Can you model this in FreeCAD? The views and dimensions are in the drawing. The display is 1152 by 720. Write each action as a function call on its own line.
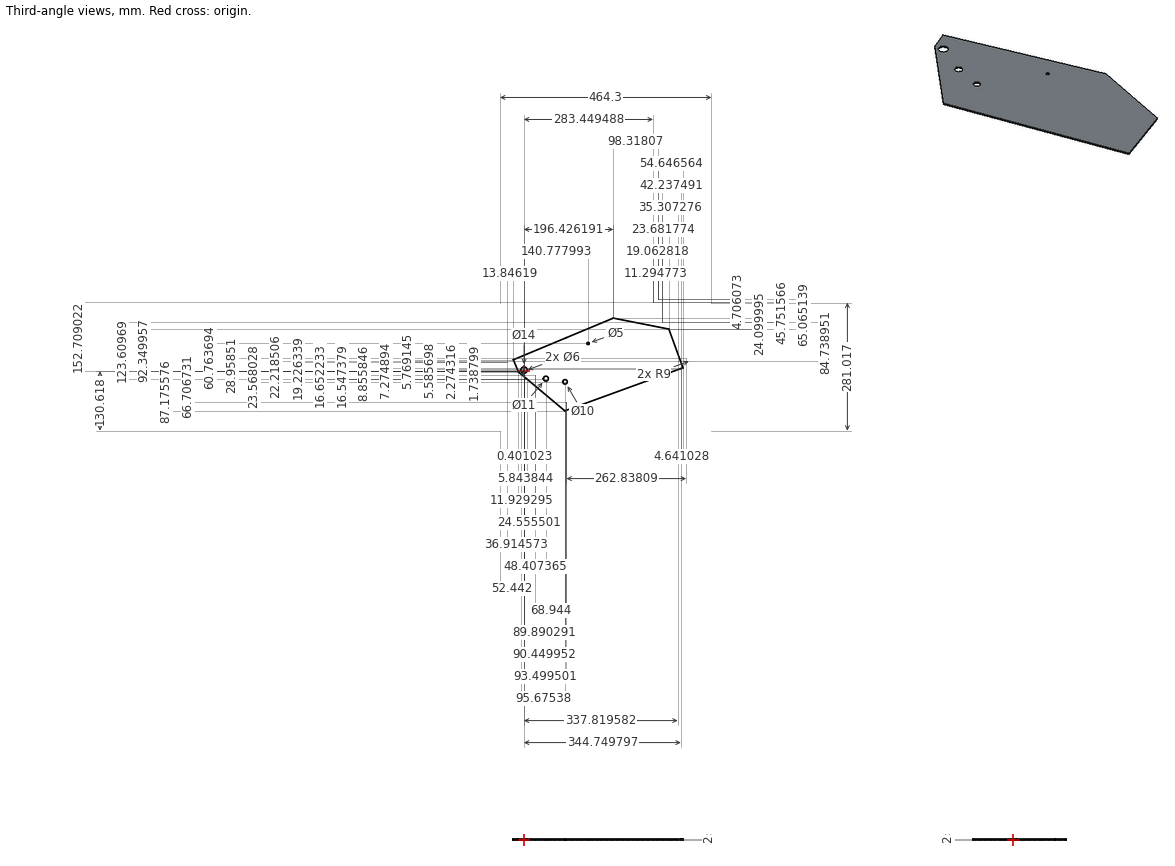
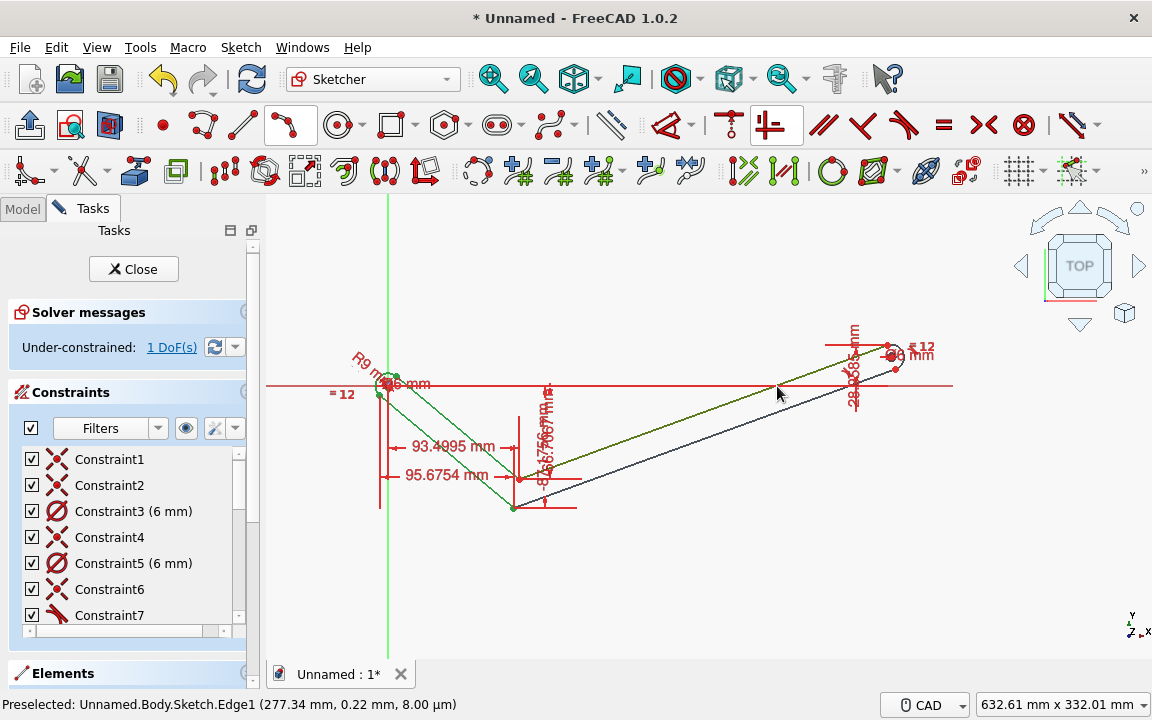
key(l)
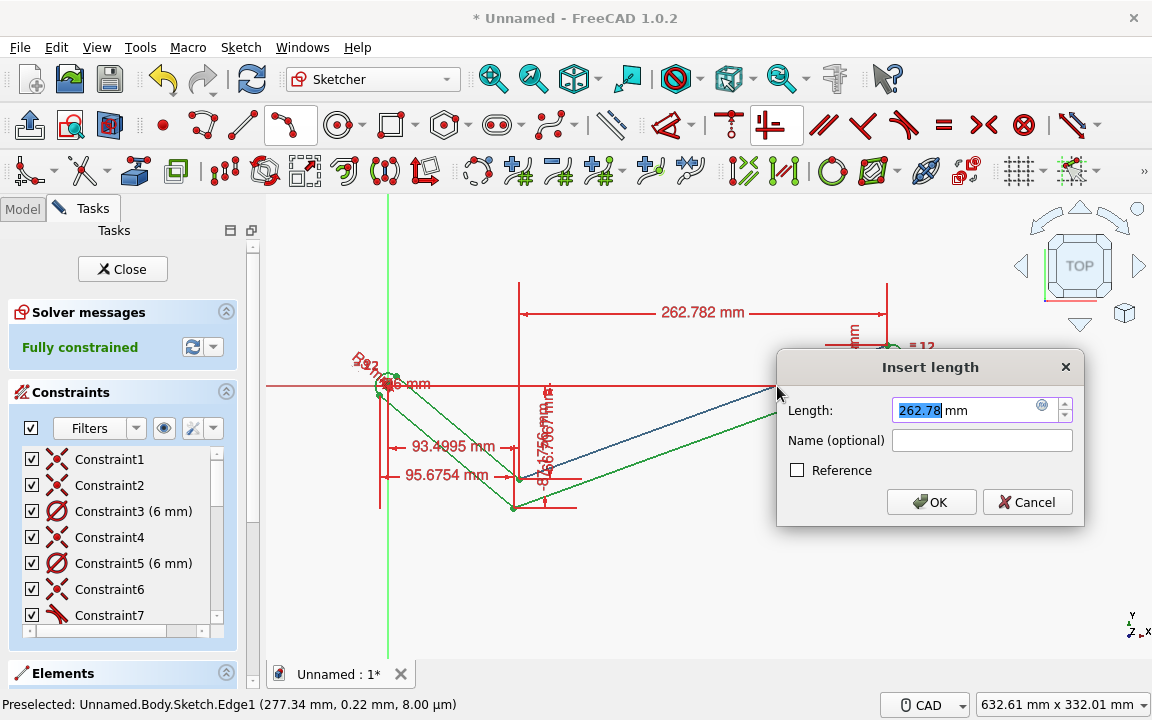
text(262.83809)
key(Return)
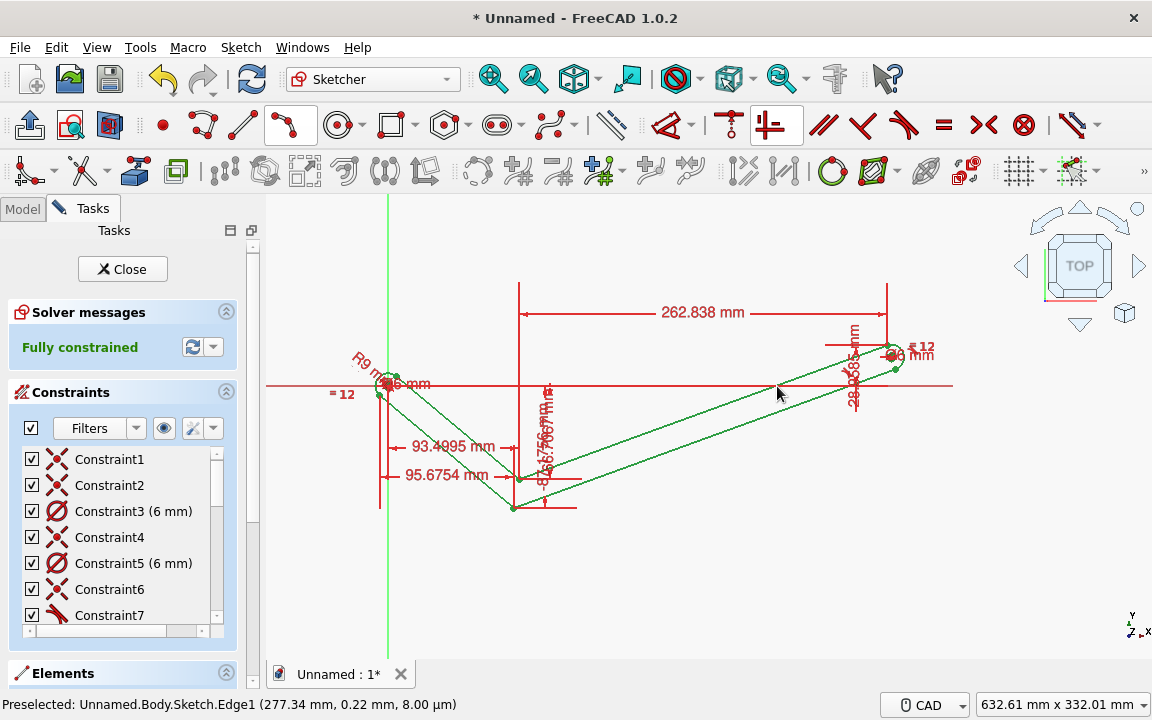
click(123, 269)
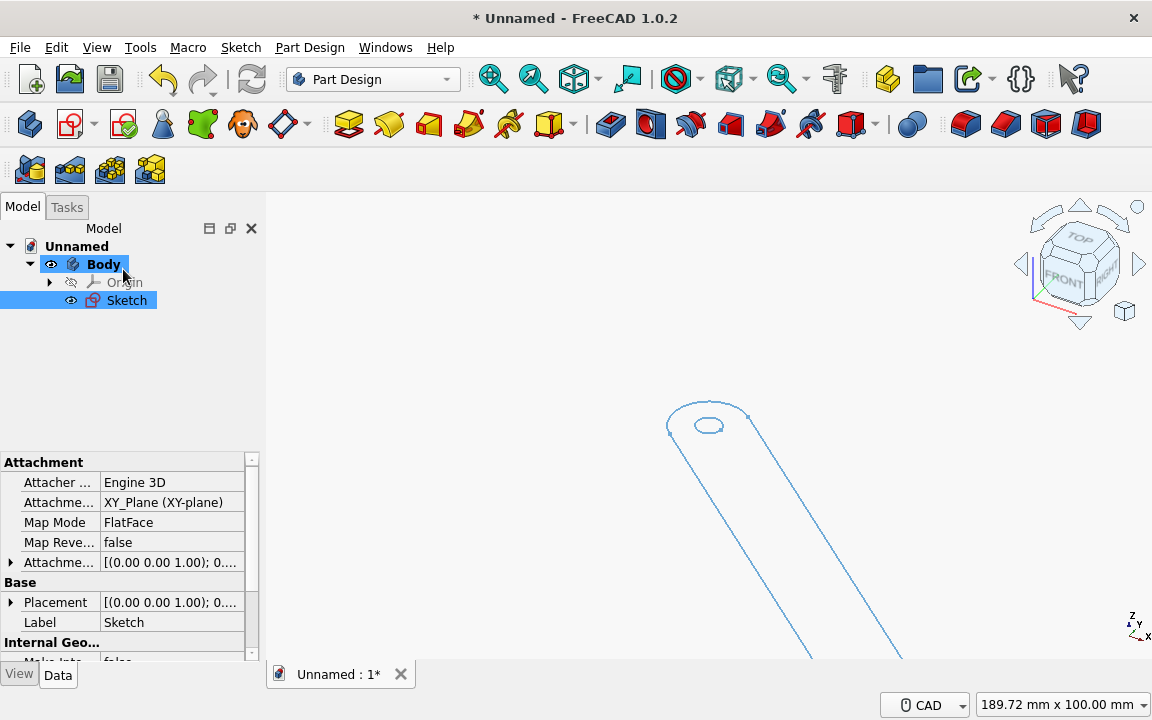
click(350, 124)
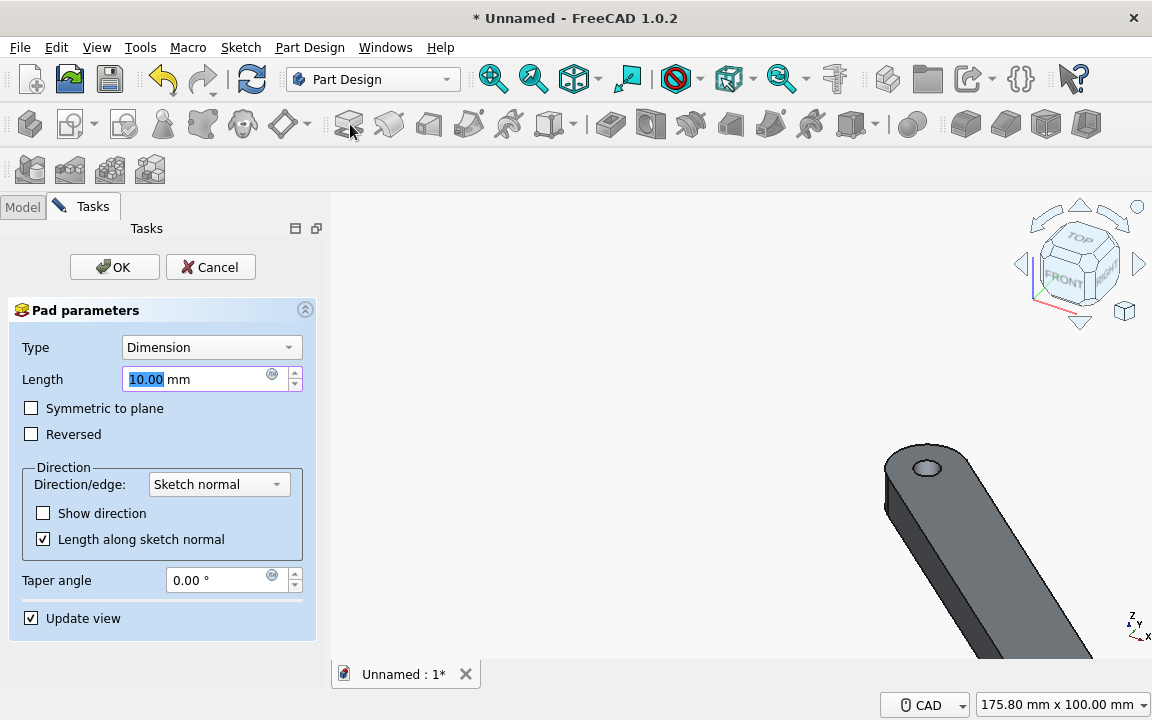
text(2)
key(Tab)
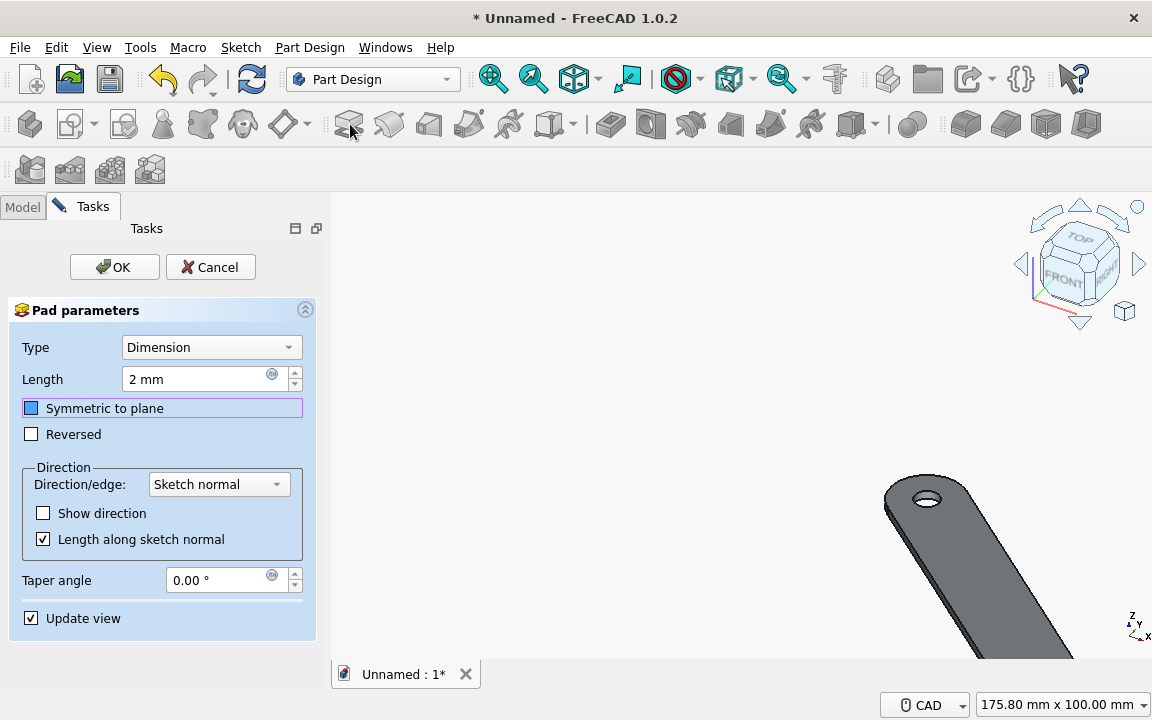
click(115, 267)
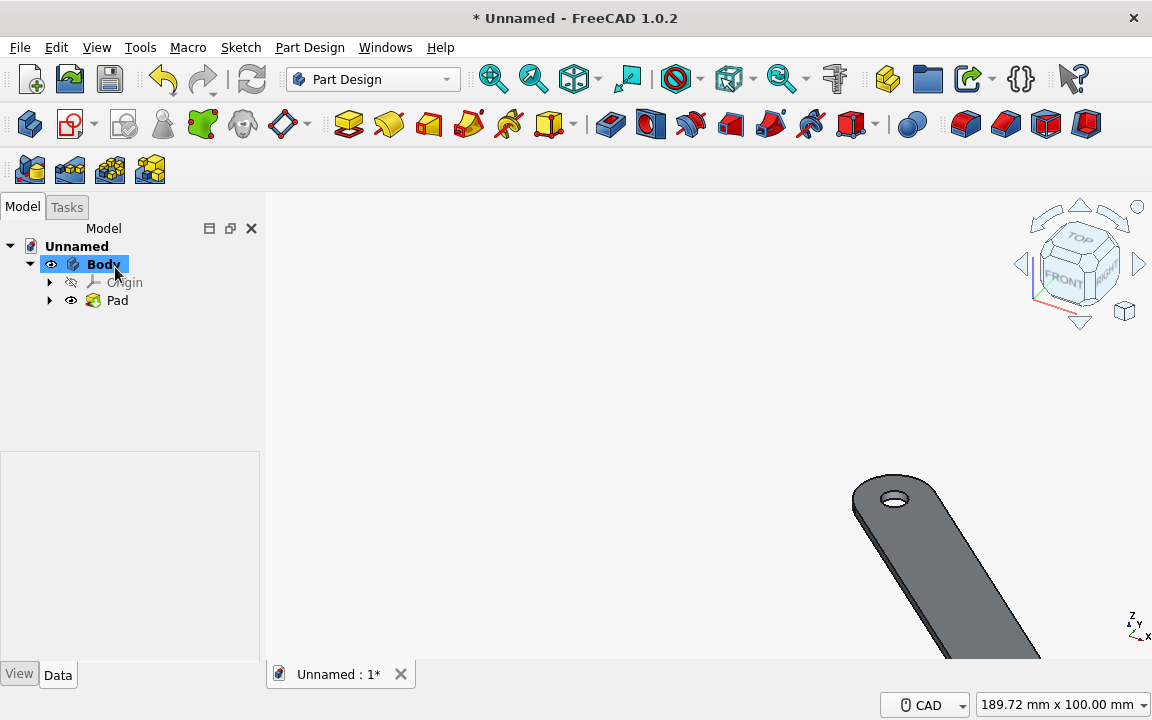
key(v)
key(f)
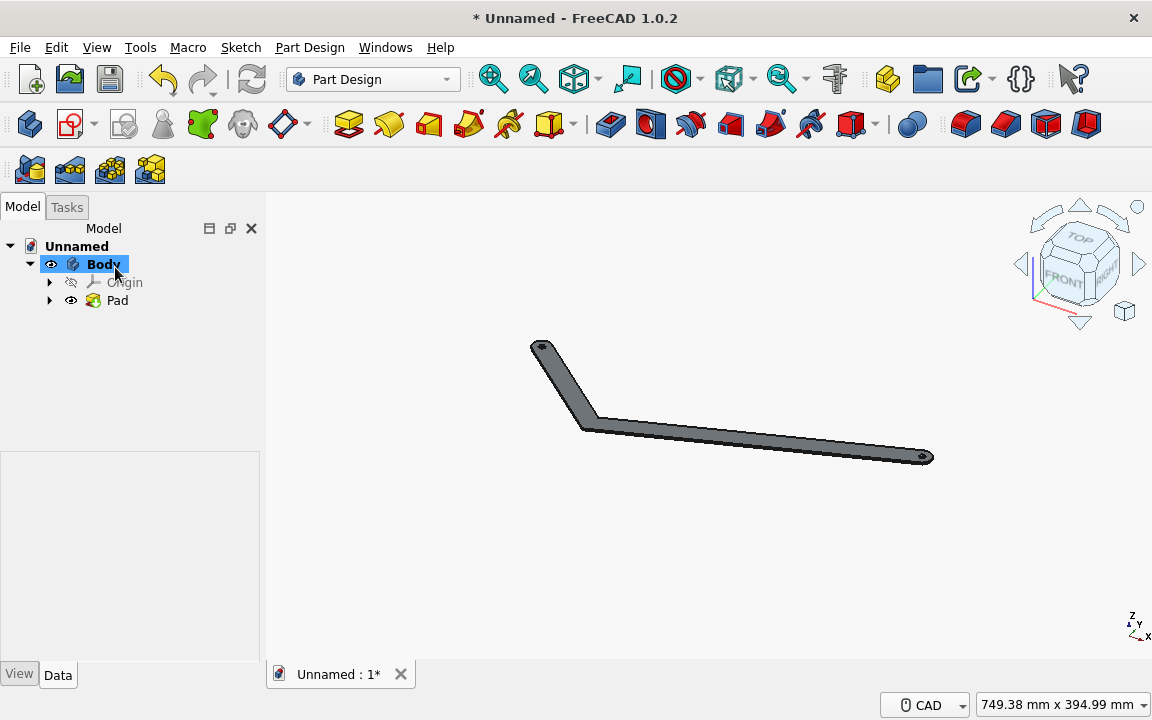
click(553, 359)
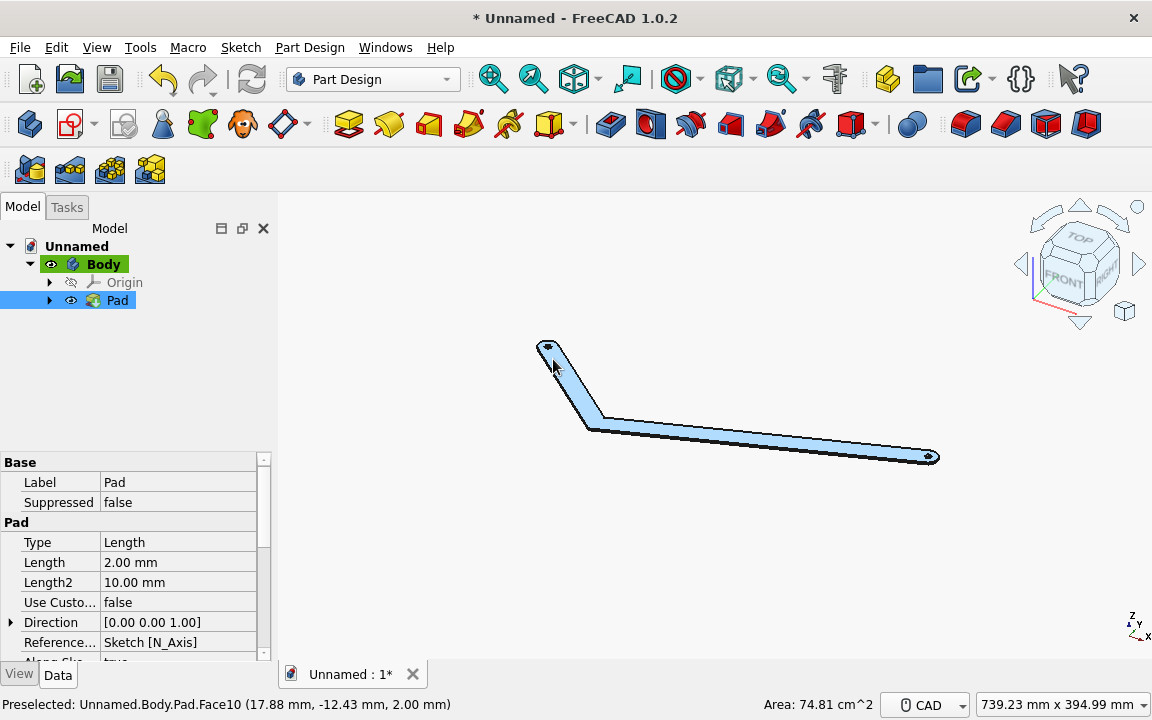
click(70, 124)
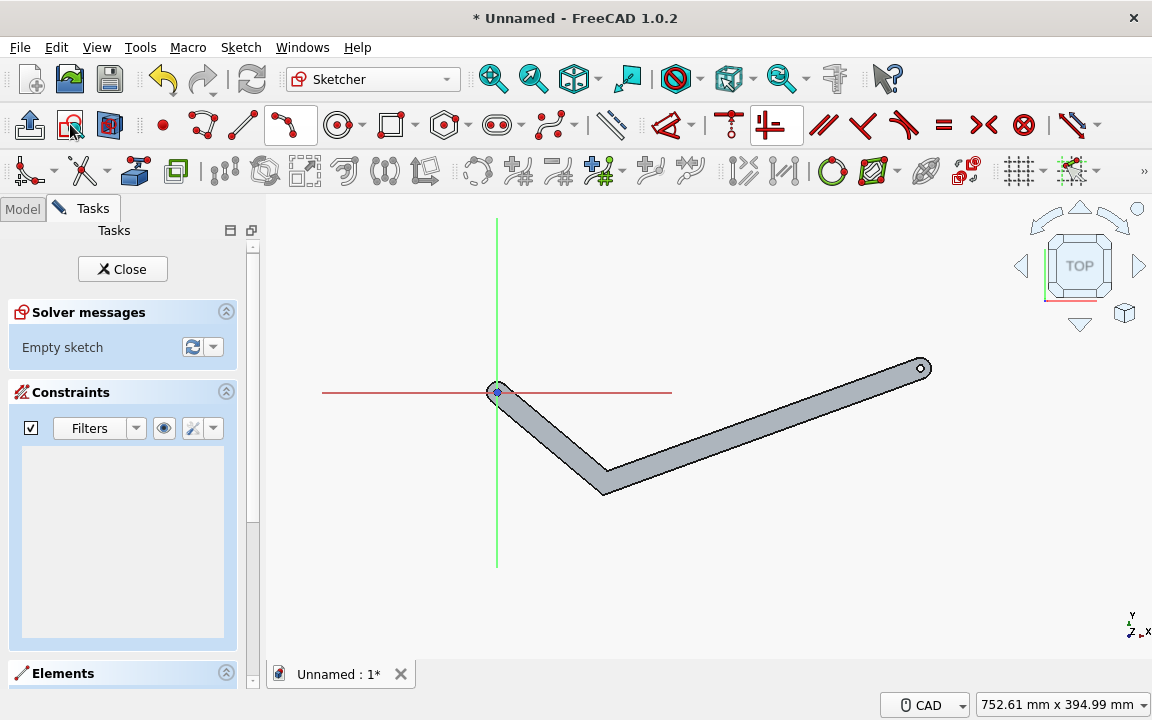
key(g)
key(m)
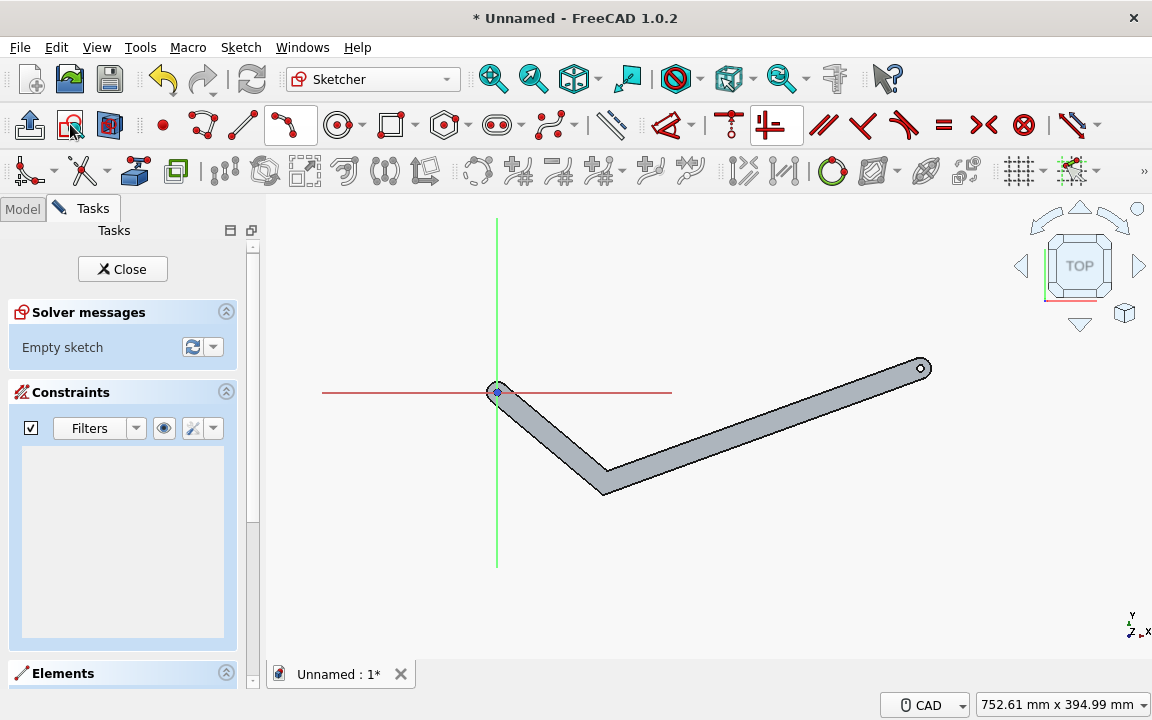
scroll(526, 403, up, 3)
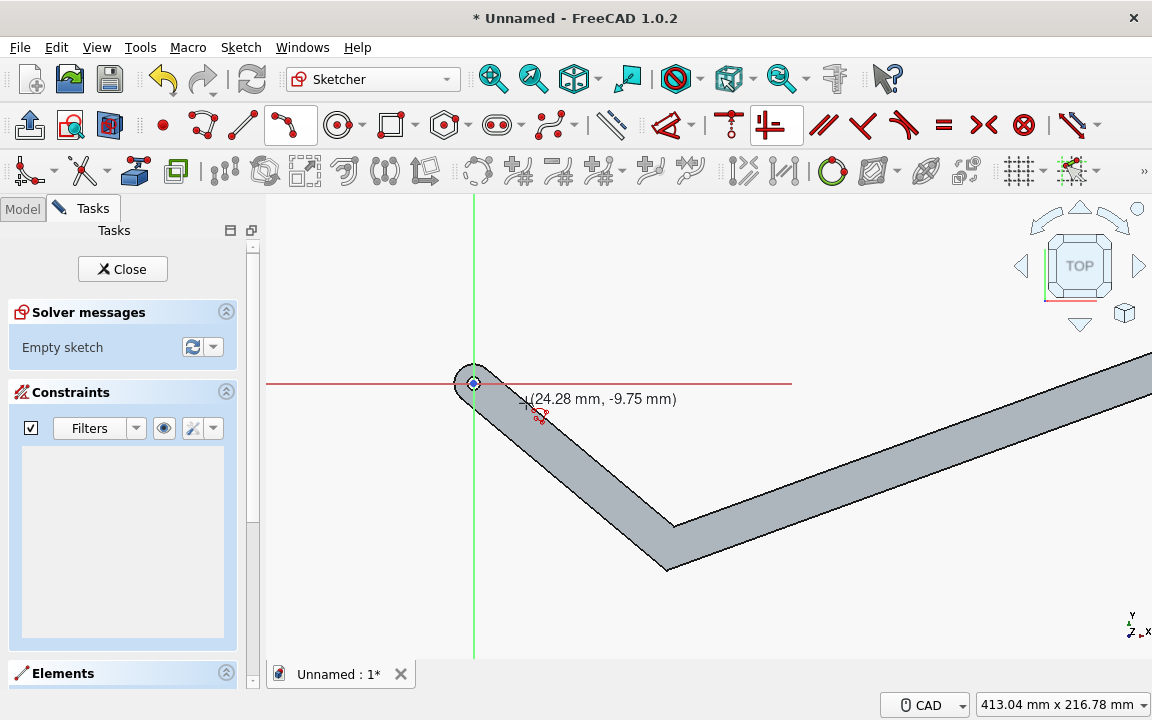
click(526, 403)
click(674, 527)